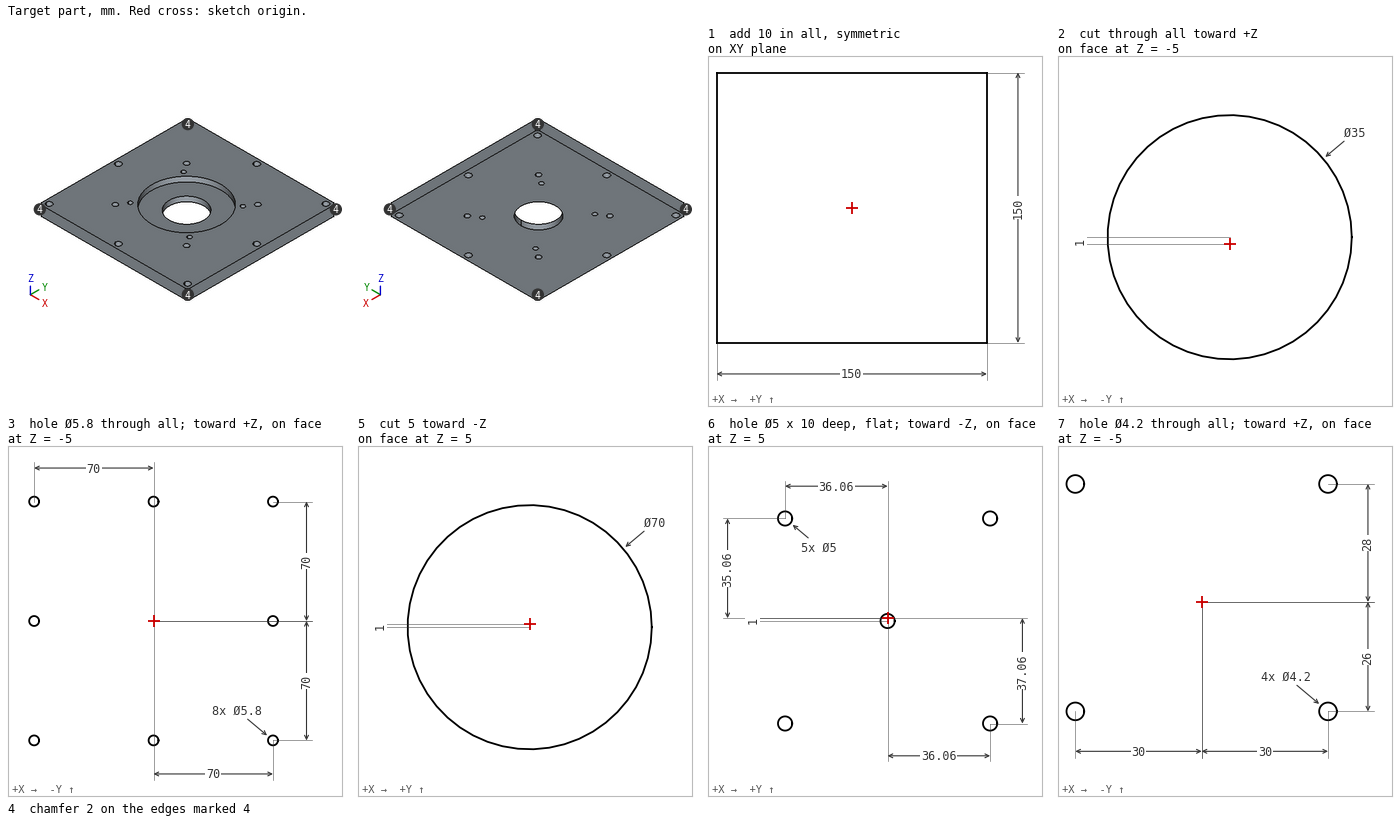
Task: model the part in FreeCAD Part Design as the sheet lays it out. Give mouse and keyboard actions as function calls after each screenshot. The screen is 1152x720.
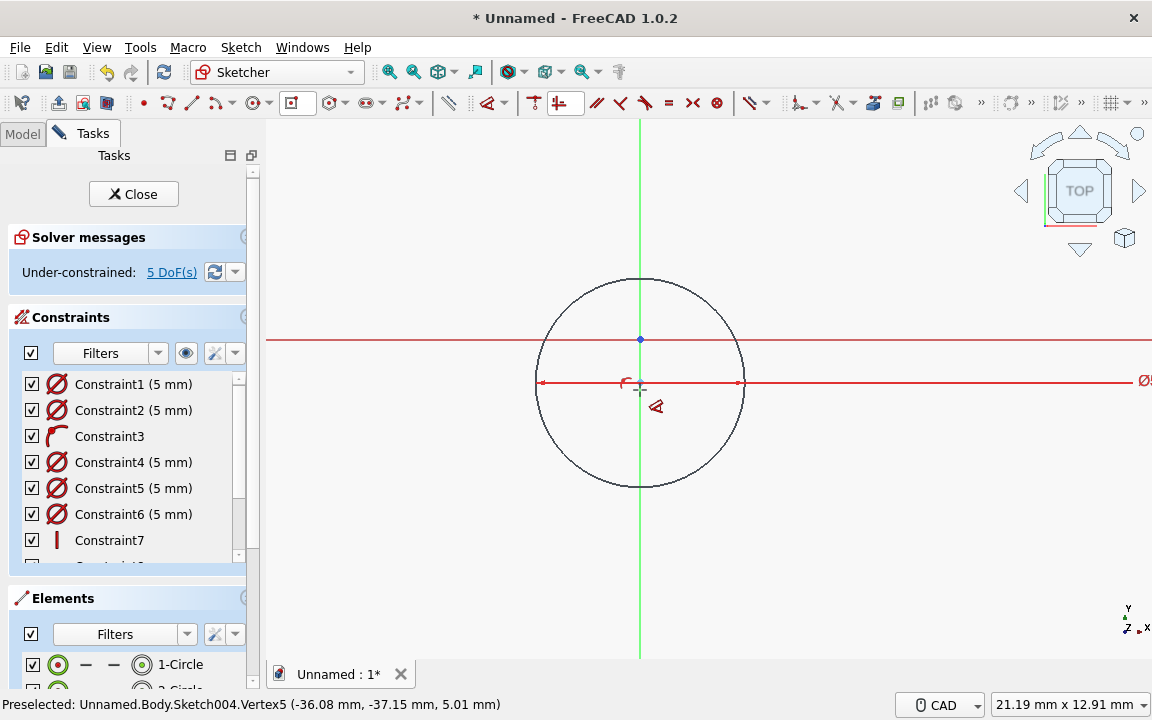
click(640, 383)
click(674, 361)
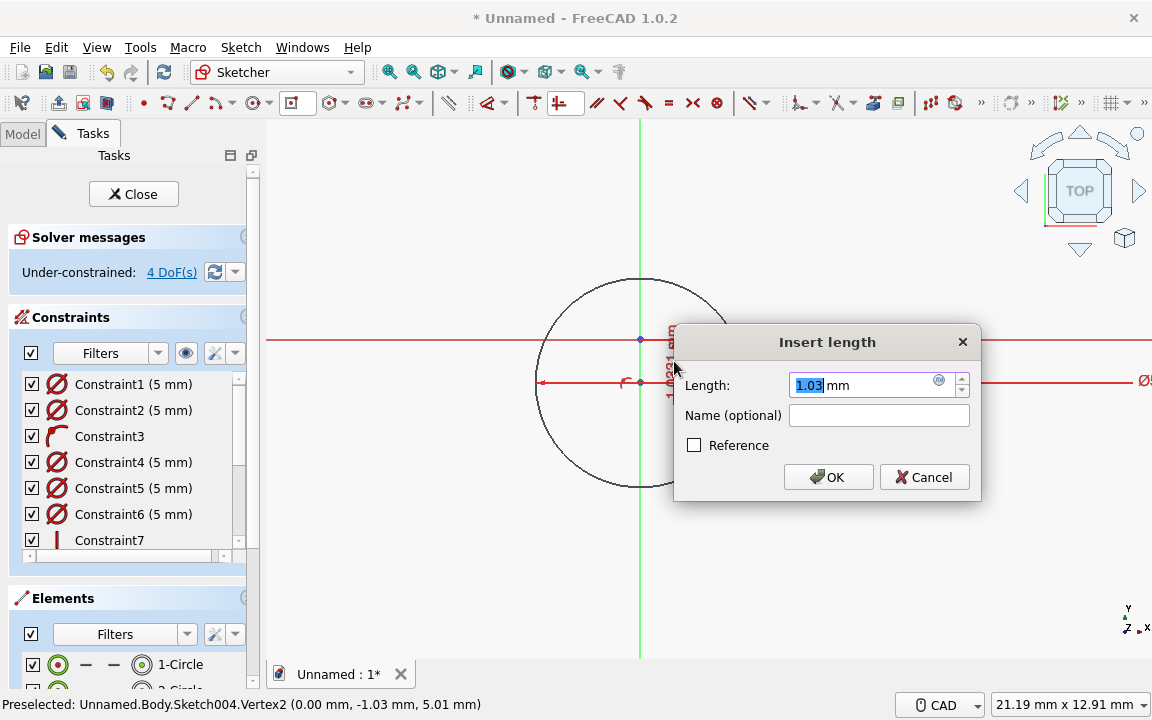
text(1)
key(Return)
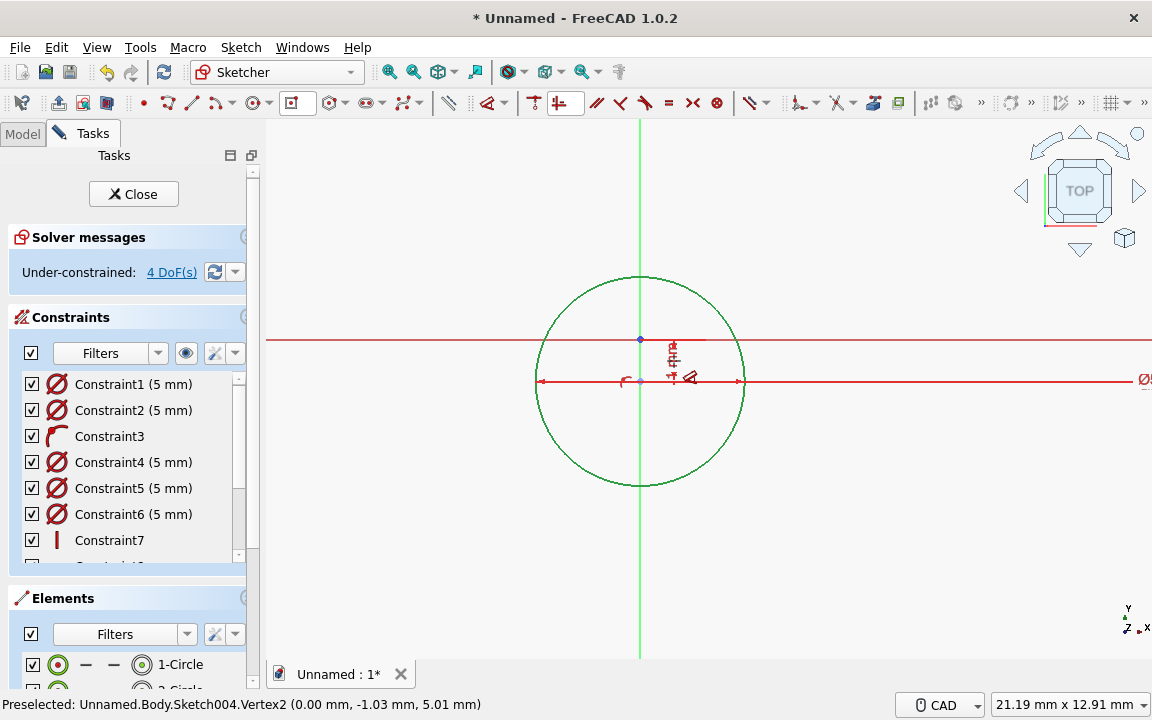
scroll(641, 390, down, 11)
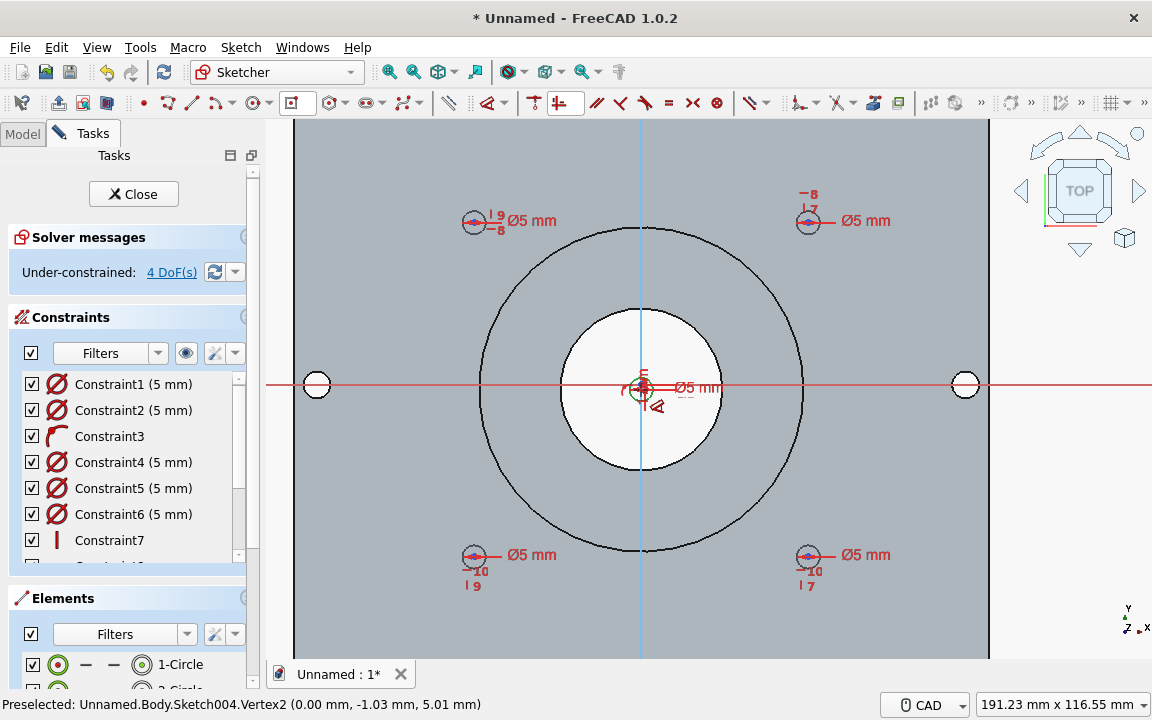
click(474, 223)
click(558, 189)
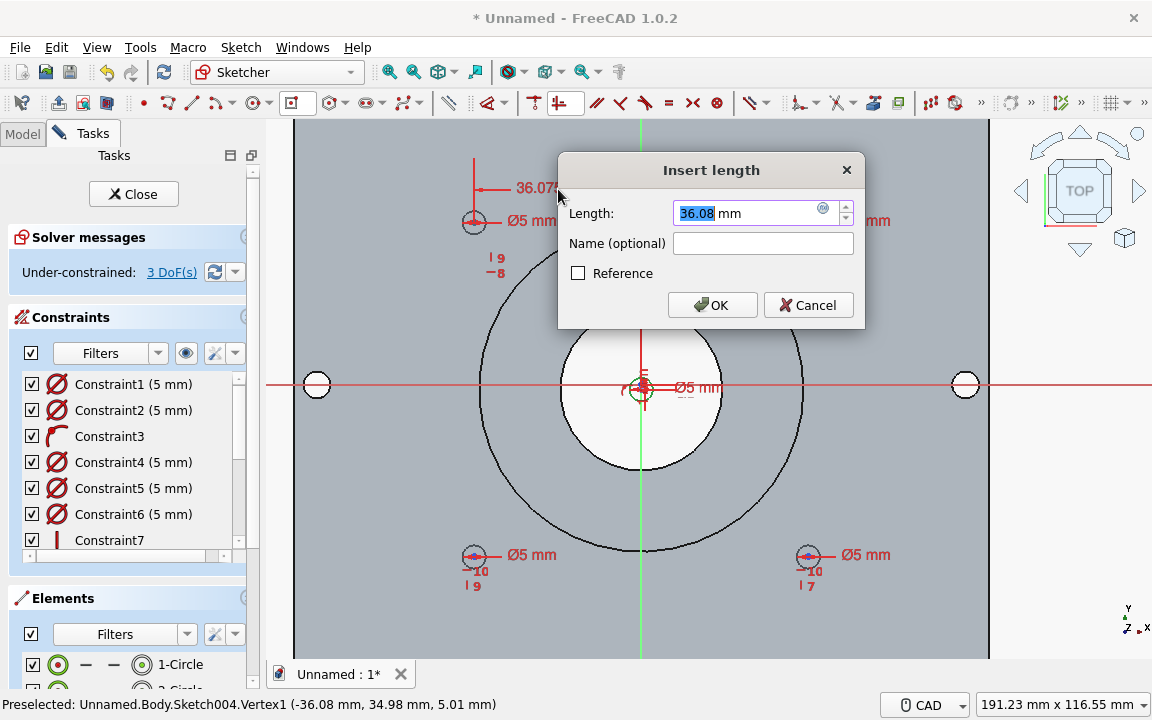
text(36.06)
key(Return)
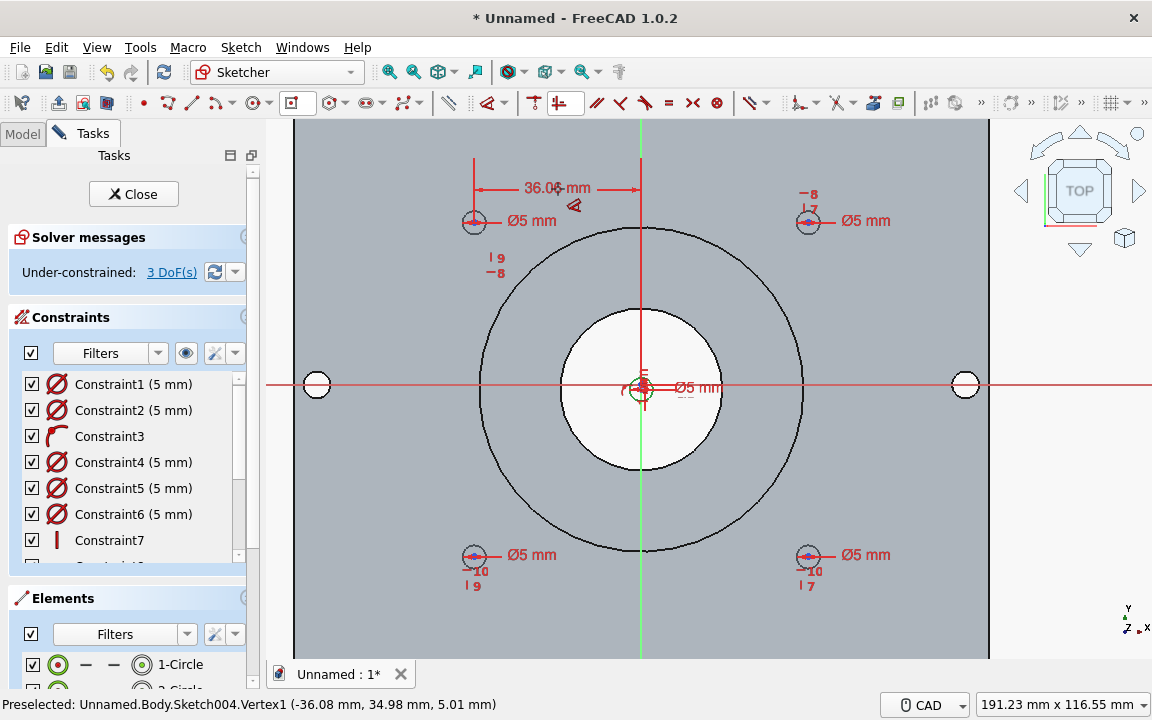
click(474, 223)
click(440, 304)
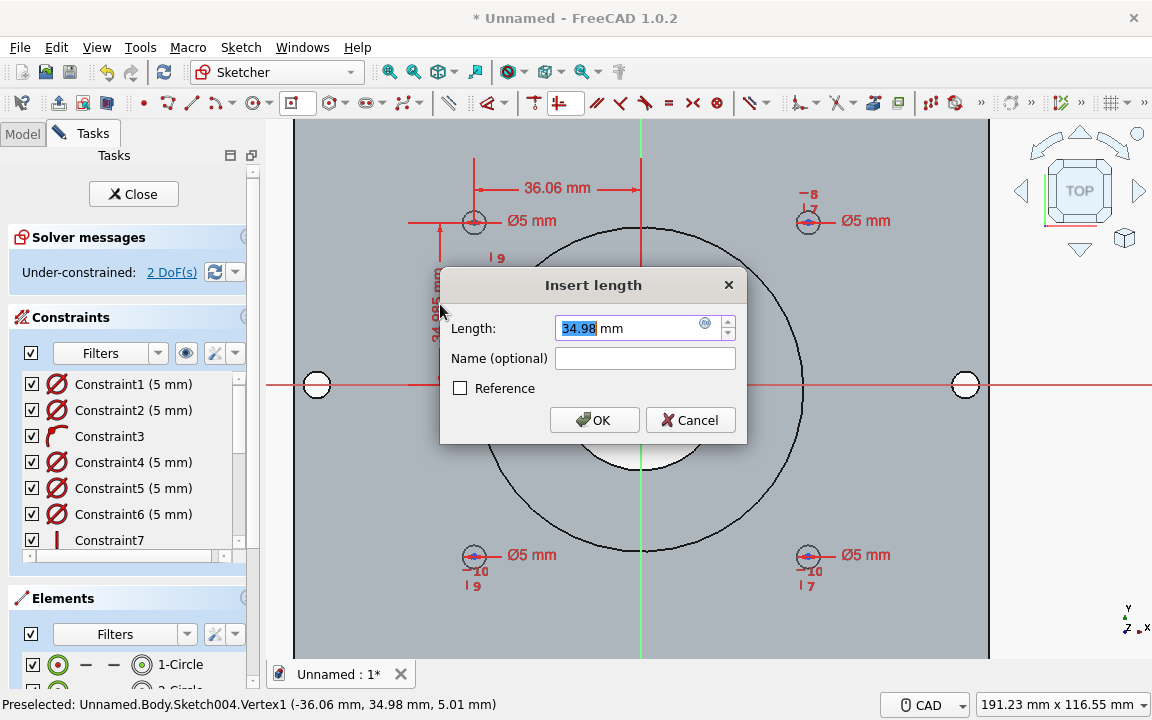
text(35.06)
key(Return)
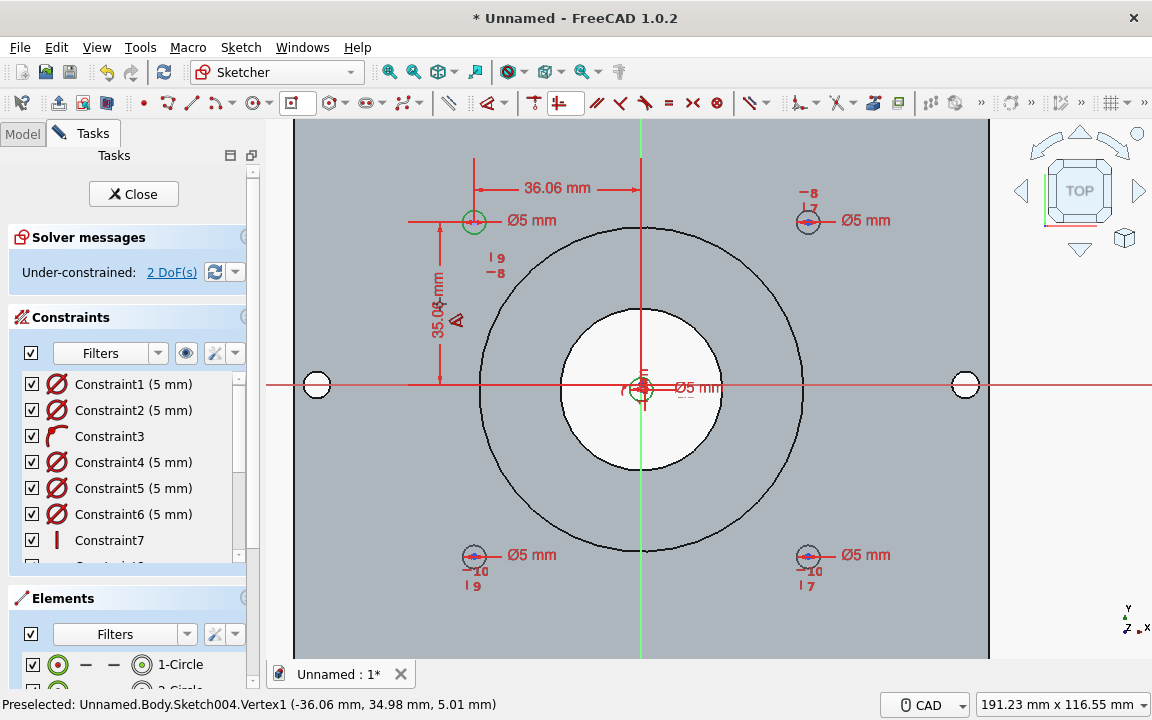
click(808, 557)
click(725, 591)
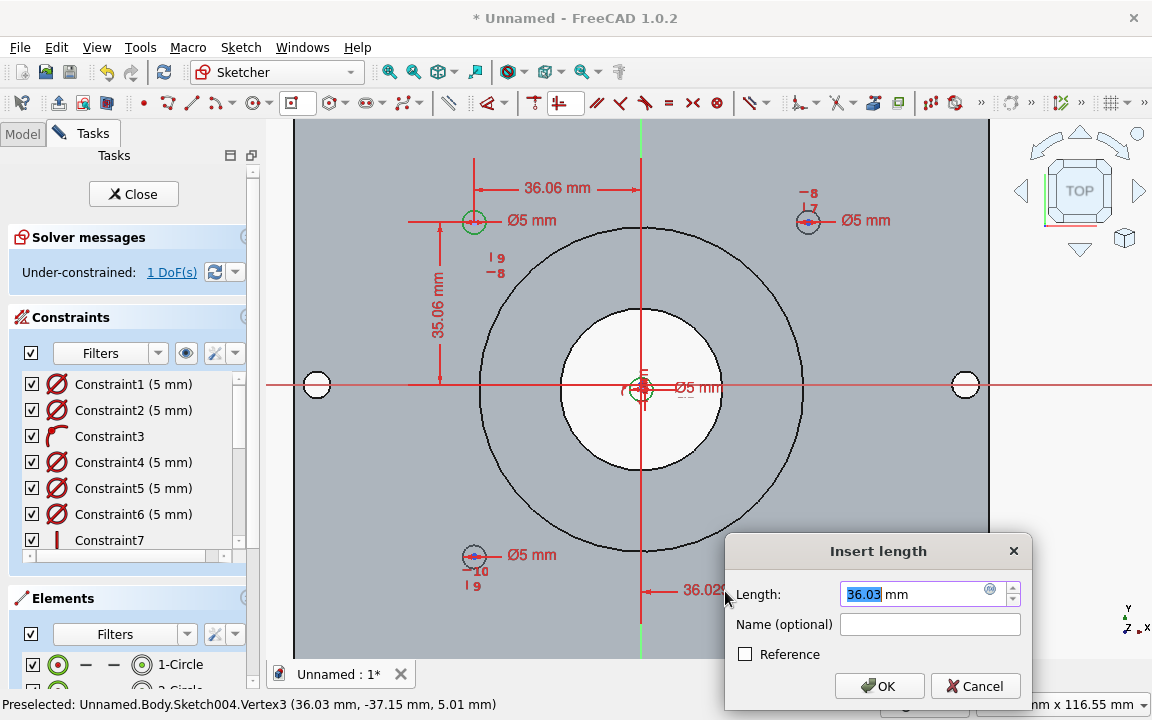
text(36.06)
key(Return)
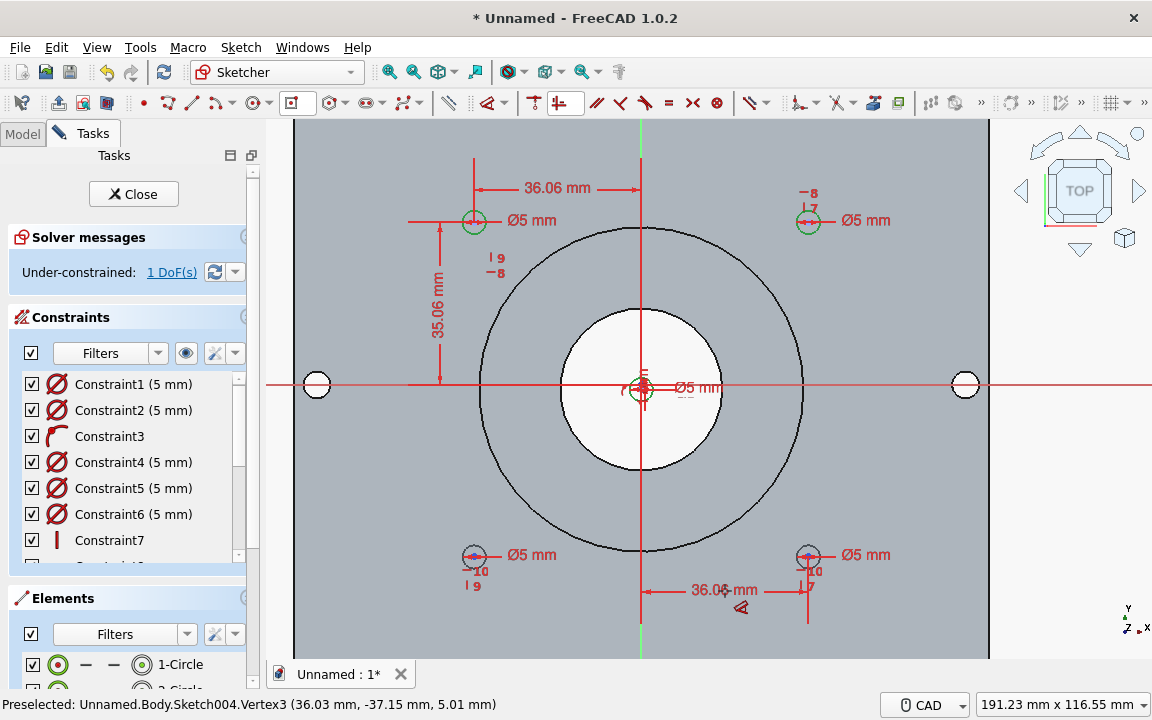
click(808, 557)
click(842, 471)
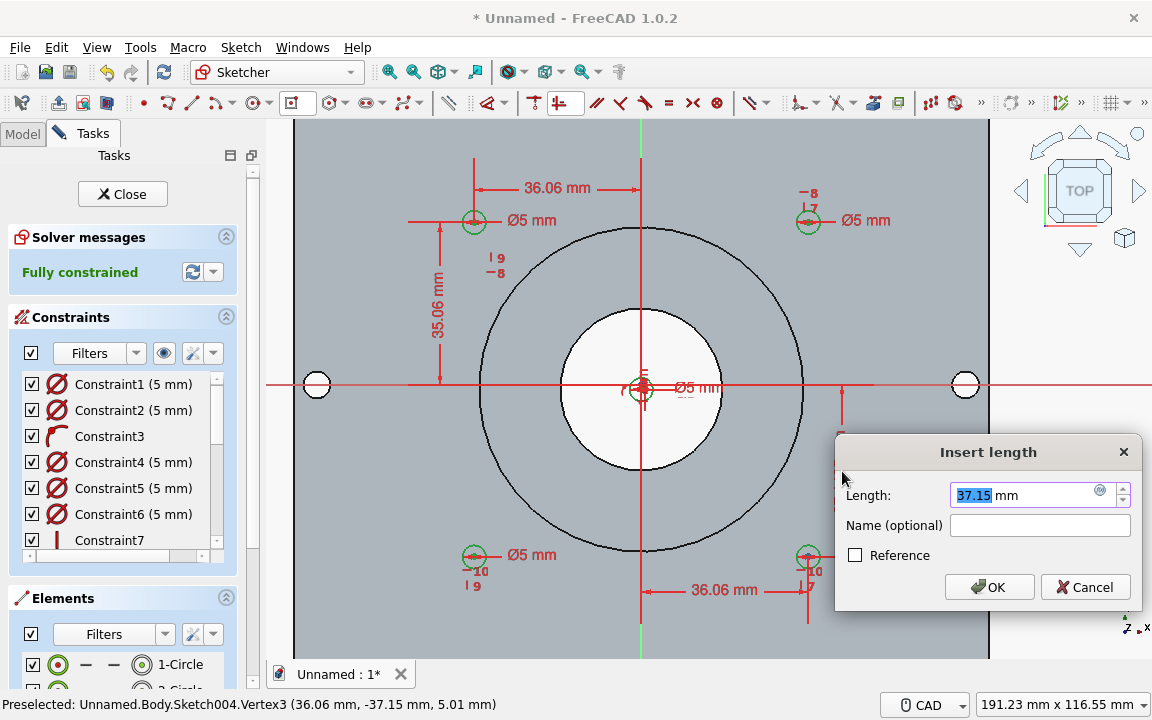
text(37.06)
key(Return)
key(Escape)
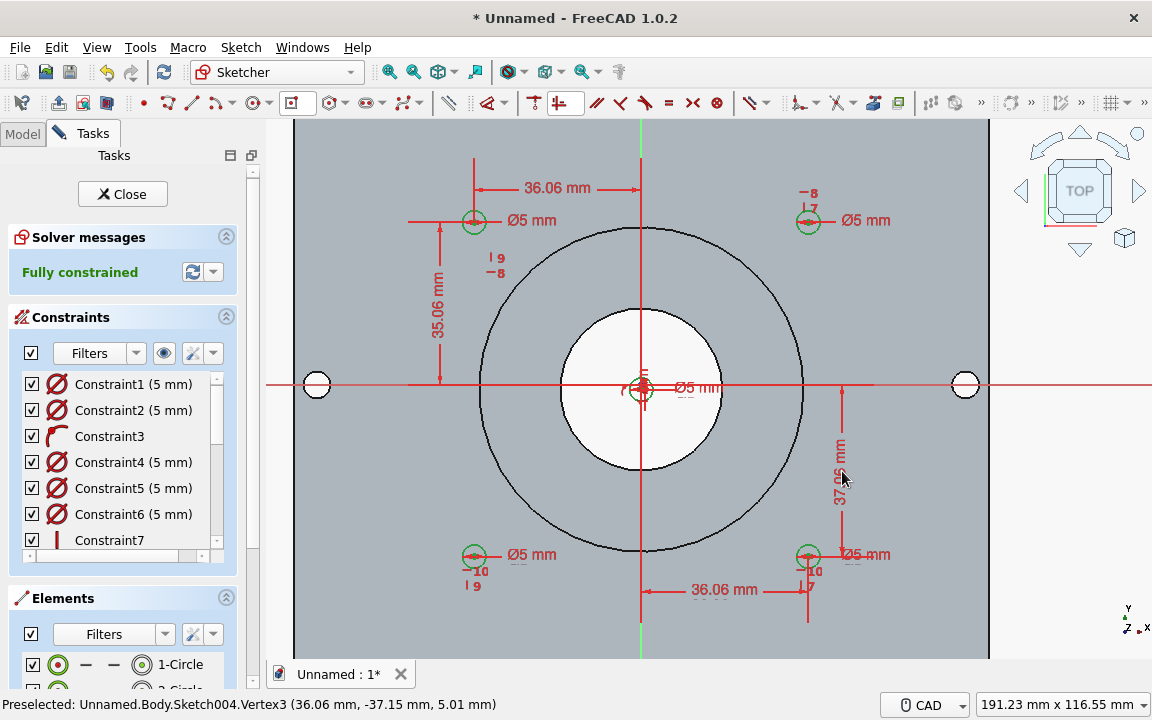
click(123, 194)